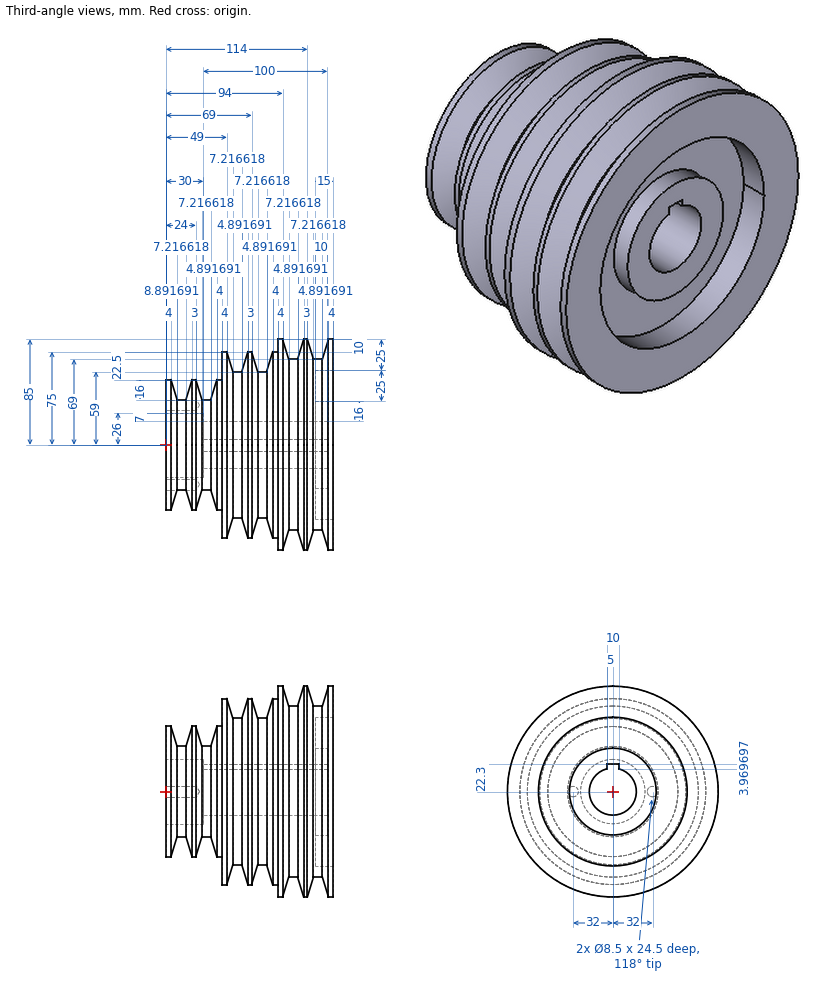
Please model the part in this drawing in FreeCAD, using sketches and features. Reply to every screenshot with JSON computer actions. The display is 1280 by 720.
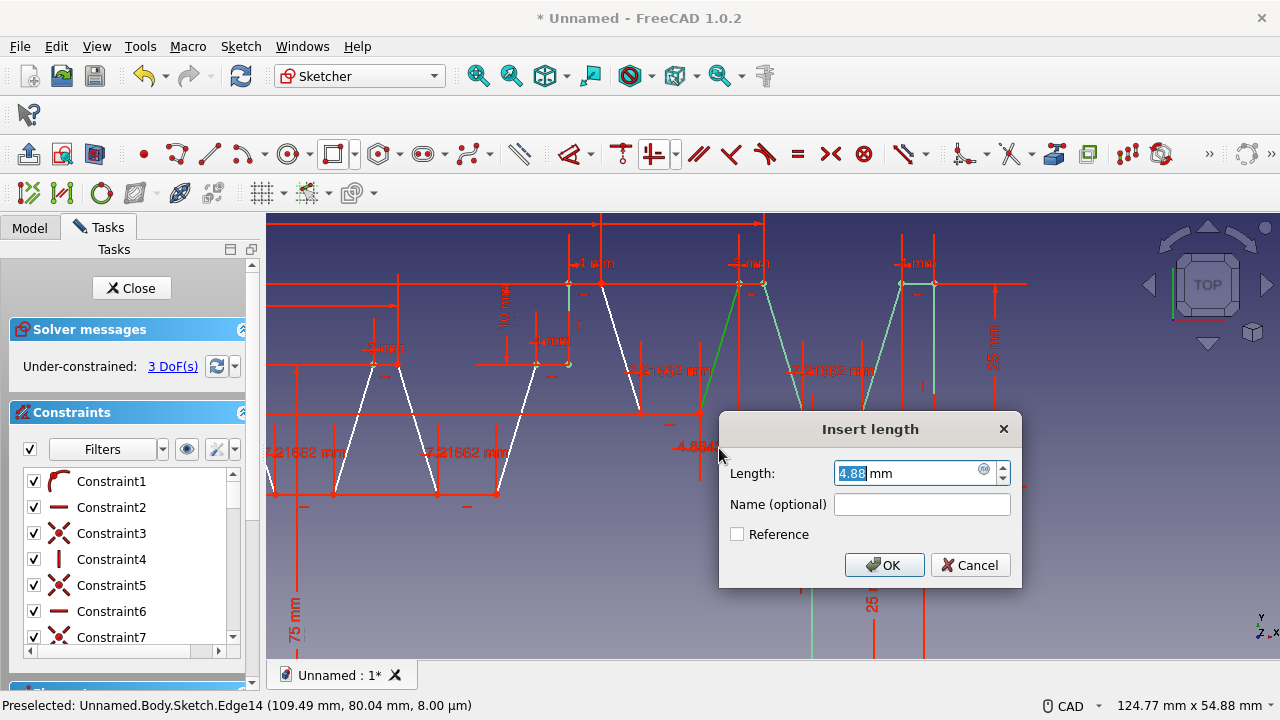
{"action": "type", "text": "4.891691"}
{"action": "key", "text": "Return"}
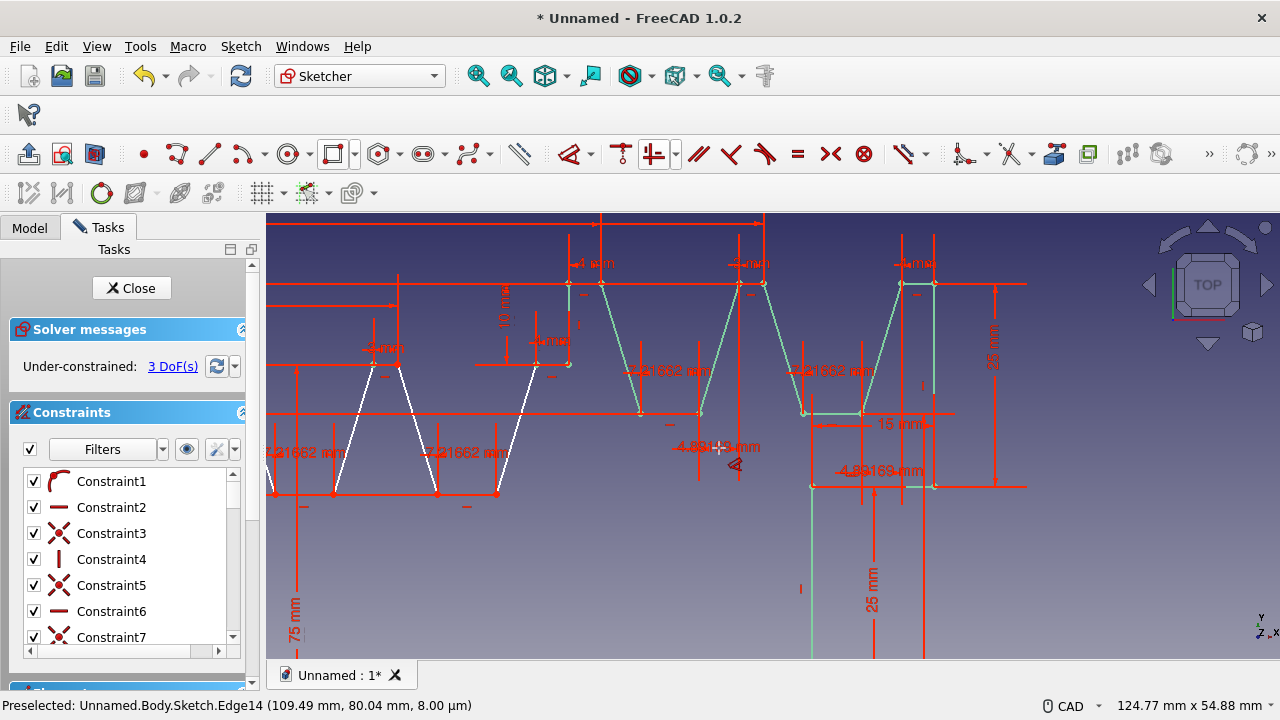
{"action": "left_click", "coordinate": [524, 404]}
{"action": "left_click", "coordinate": [516, 529]}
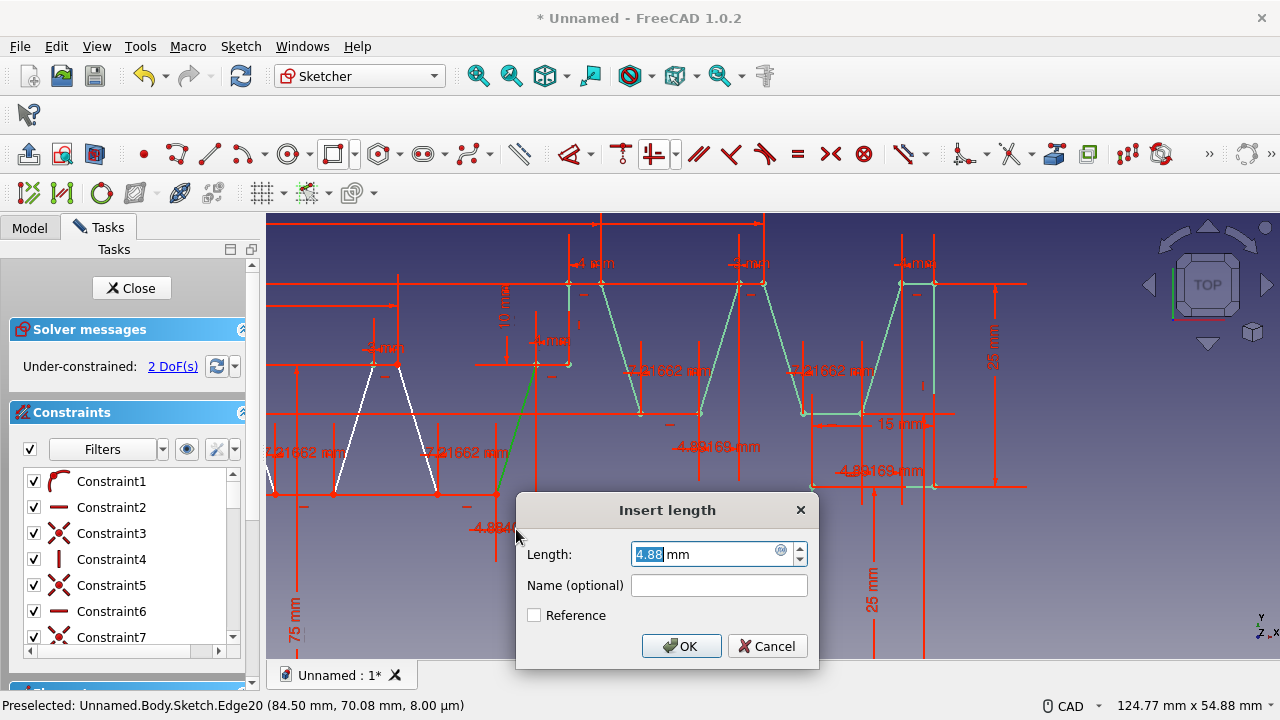
{"action": "type", "text": "4.891691"}
{"action": "key", "text": "Return"}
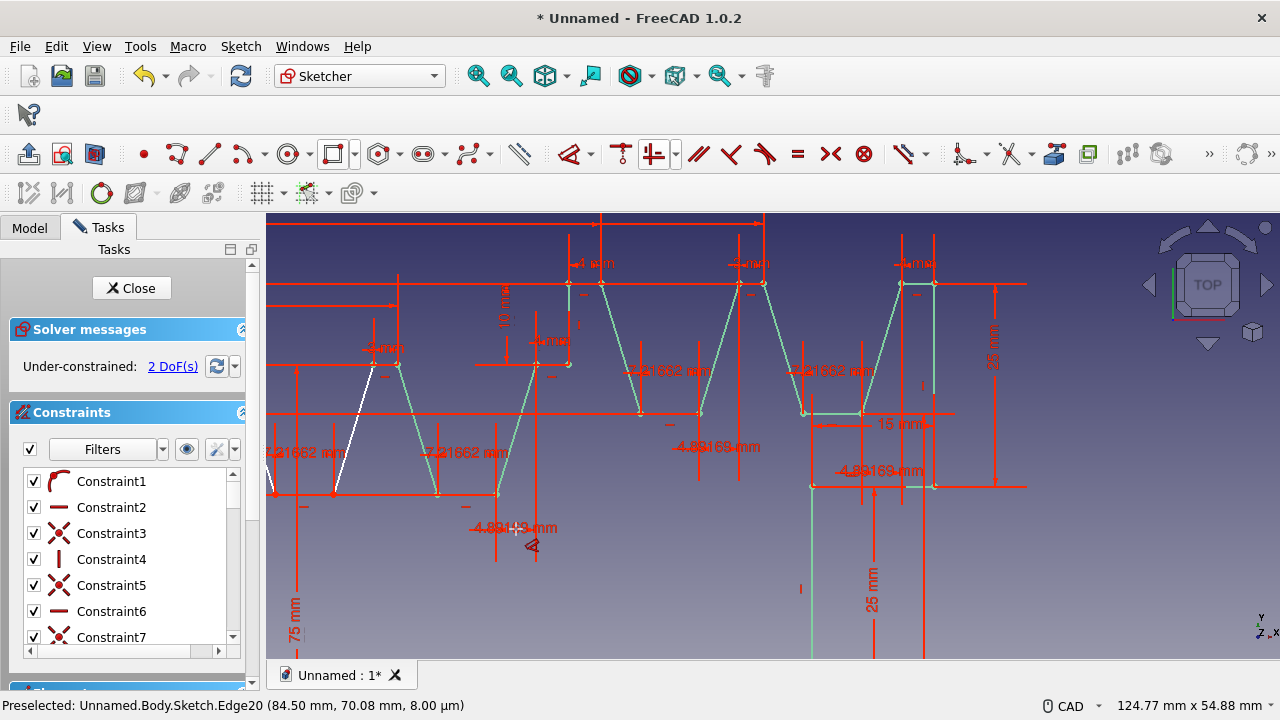
{"action": "left_click", "coordinate": [362, 404]}
{"action": "left_click", "coordinate": [354, 331]}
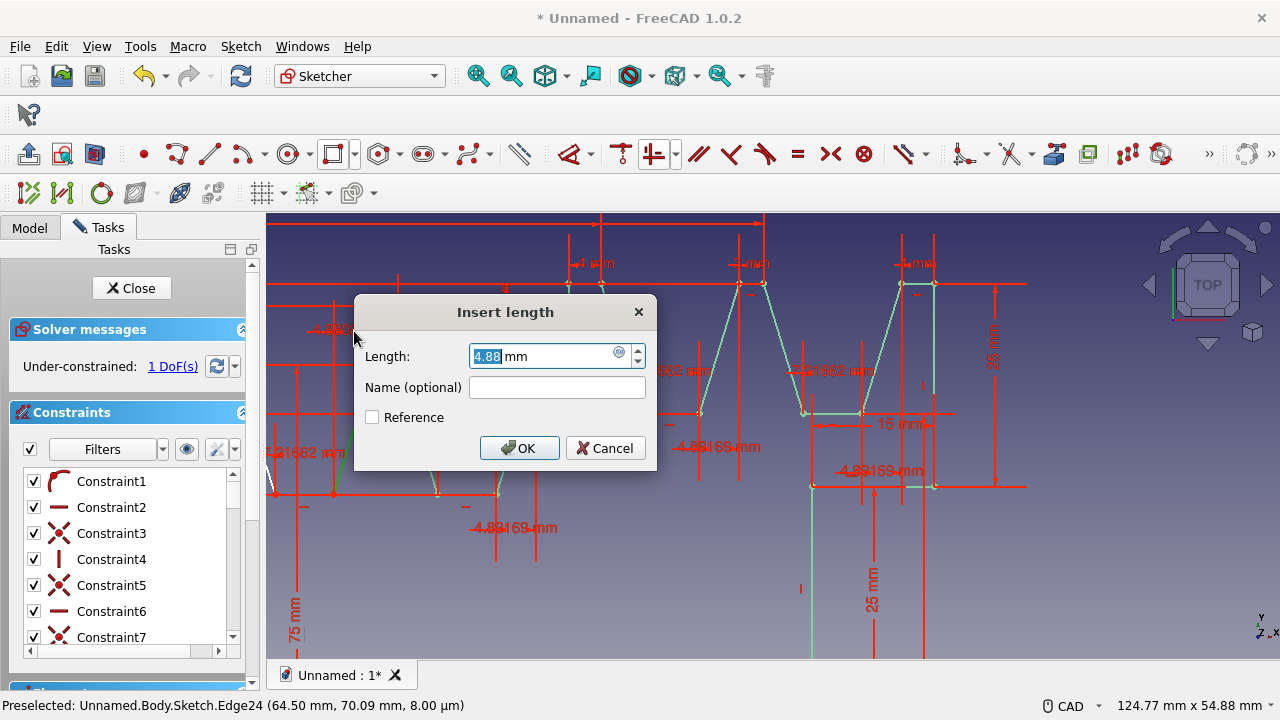
{"action": "type", "text": "4.891691"}
{"action": "key", "text": "Return"}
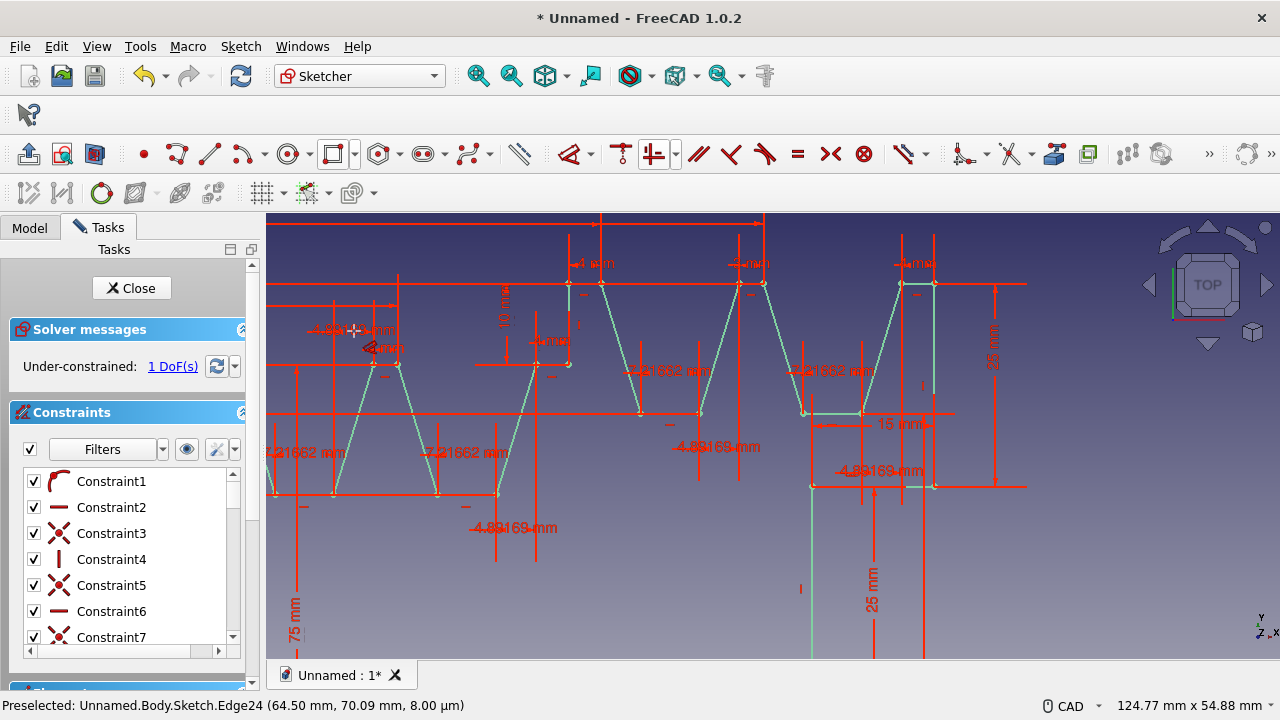
{"action": "scroll", "coordinate": [890, 324], "scroll_direction": "down", "scroll_amount": 5}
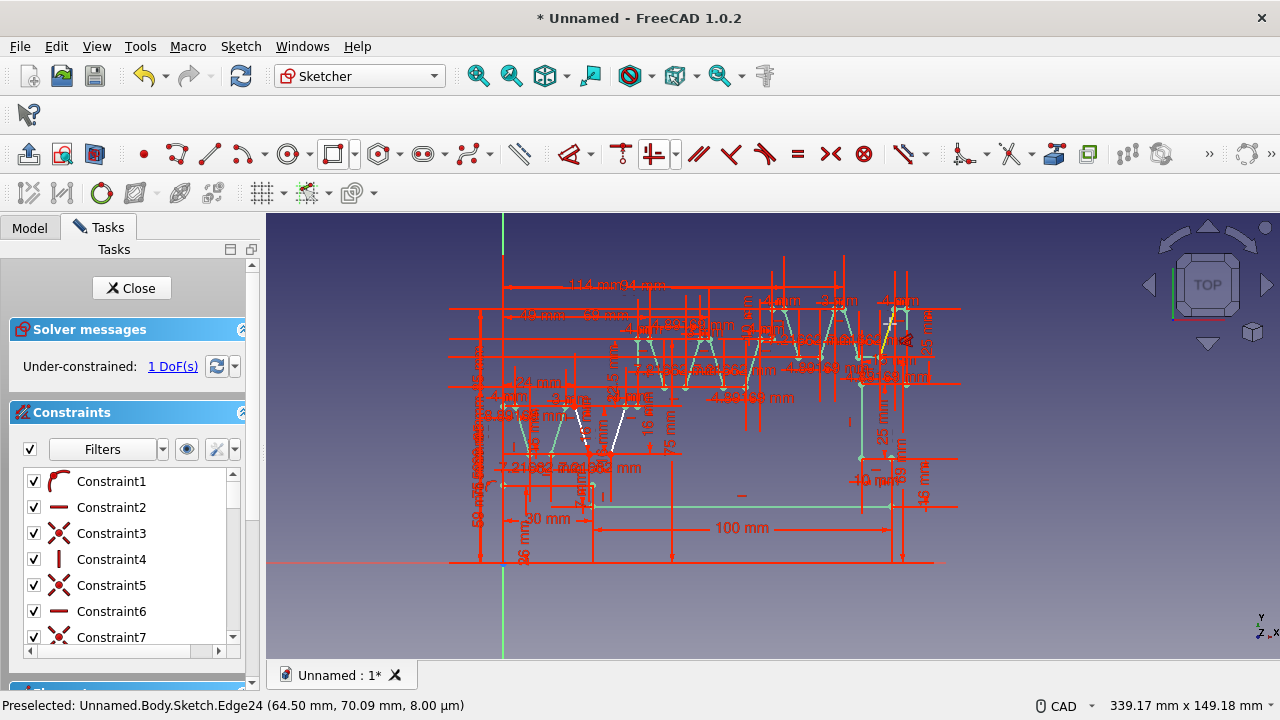
{"action": "scroll", "coordinate": [621, 421], "scroll_direction": "up", "scroll_amount": 5}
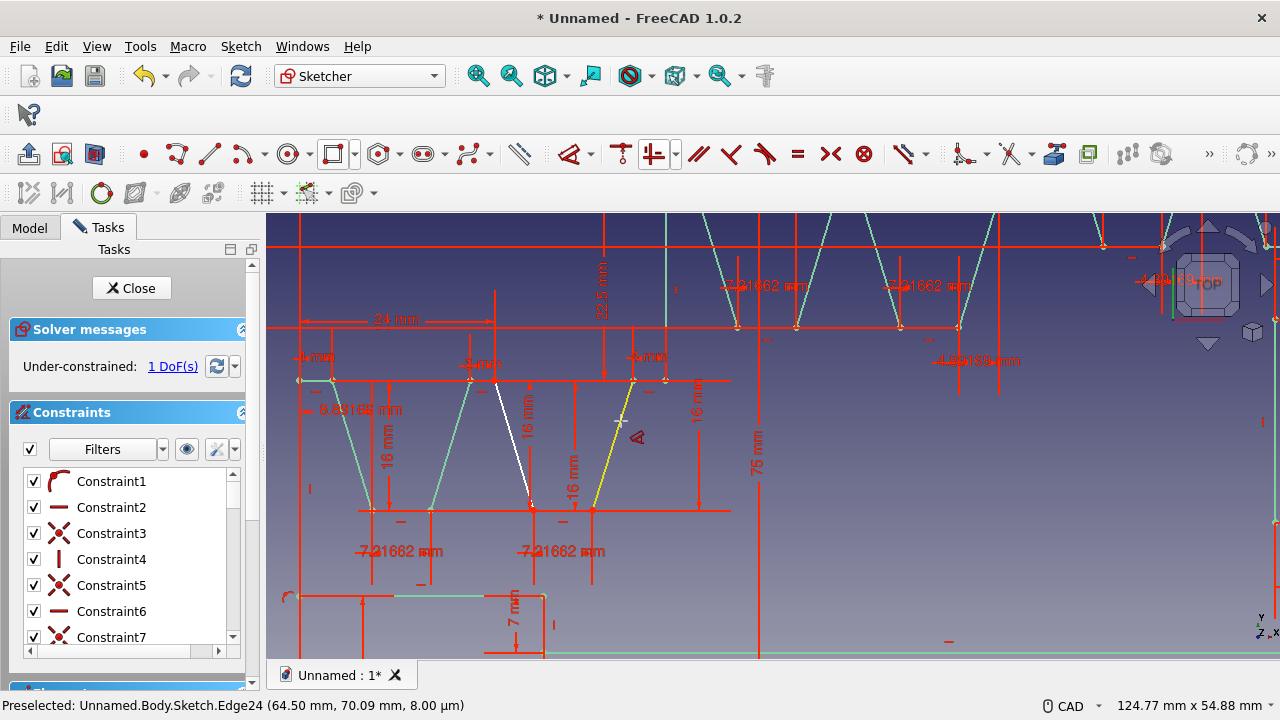
{"action": "left_click", "coordinate": [621, 420]}
{"action": "left_click", "coordinate": [613, 323]}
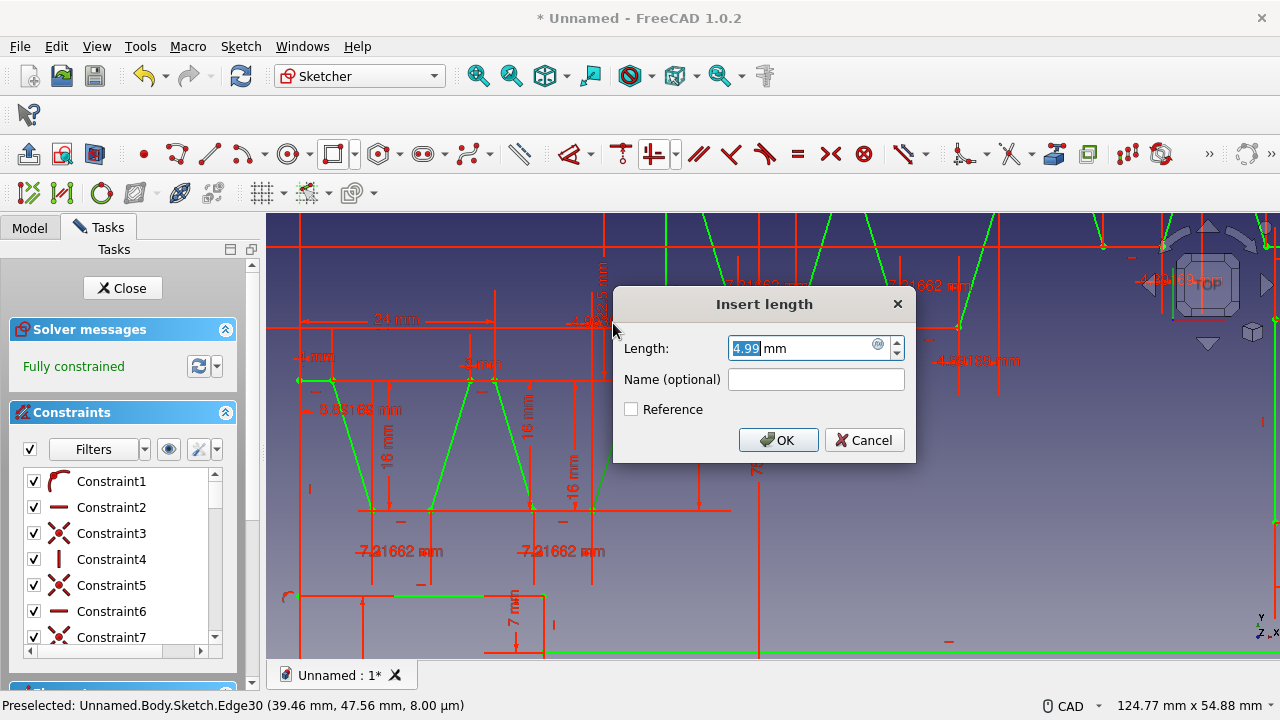
{"action": "type", "text": "4.891691"}
{"action": "key", "text": "Return"}
{"action": "key", "text": "Escape"}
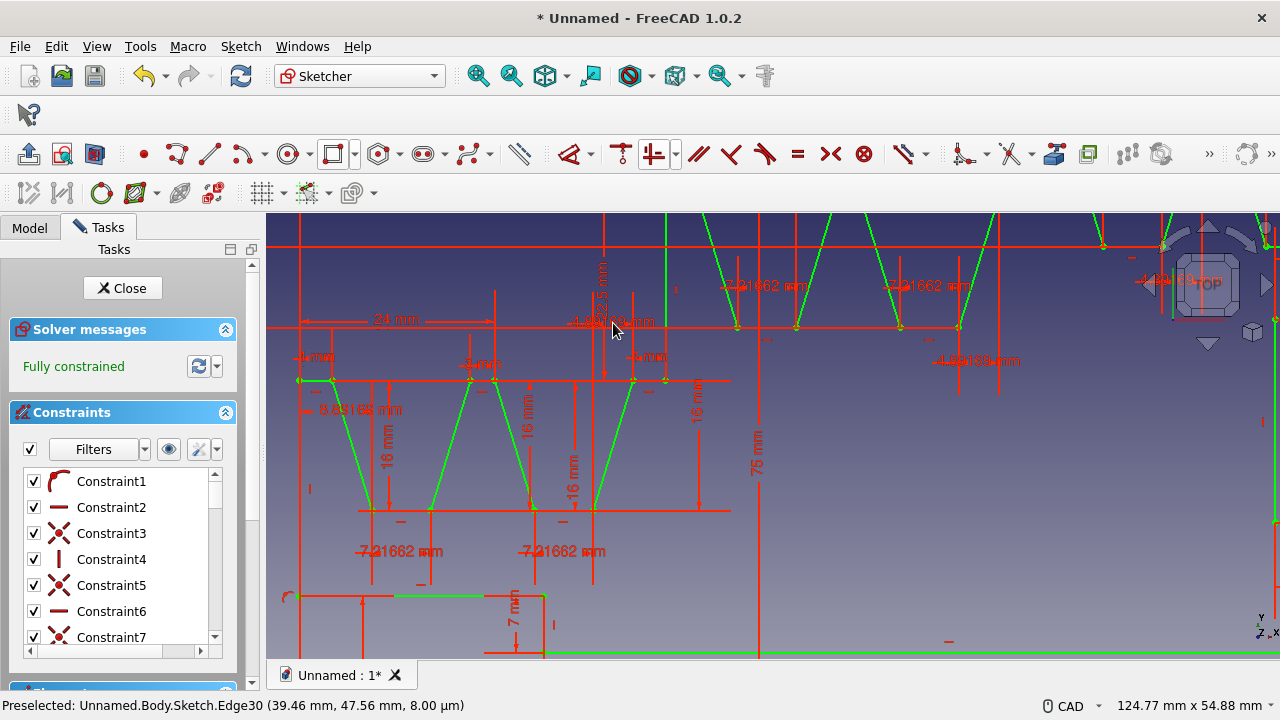
{"action": "left_click", "coordinate": [123, 288]}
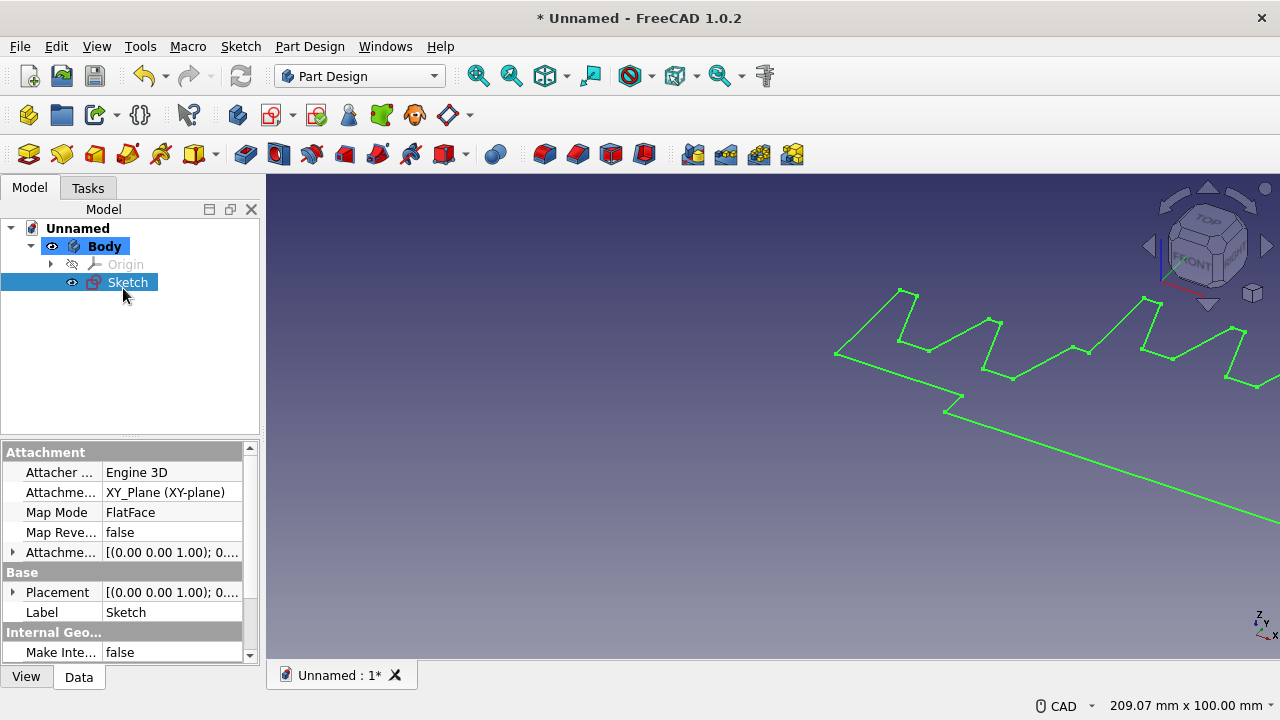
{"action": "left_click", "coordinate": [62, 154]}